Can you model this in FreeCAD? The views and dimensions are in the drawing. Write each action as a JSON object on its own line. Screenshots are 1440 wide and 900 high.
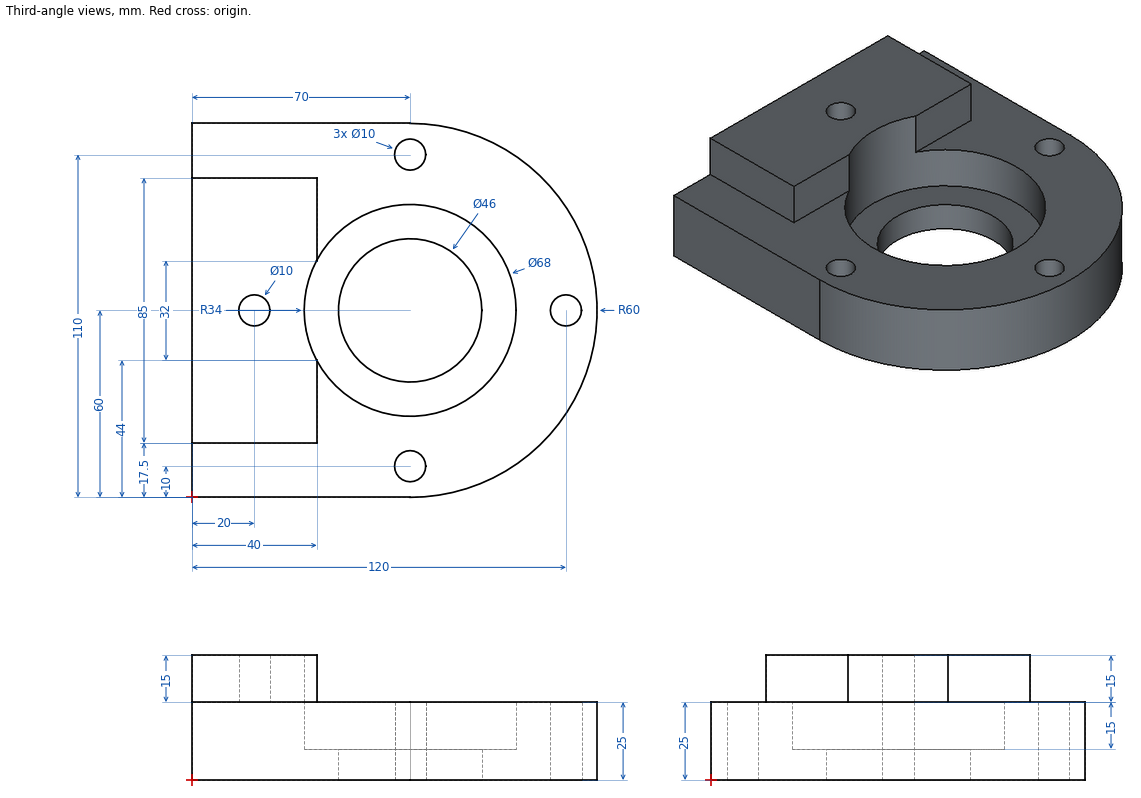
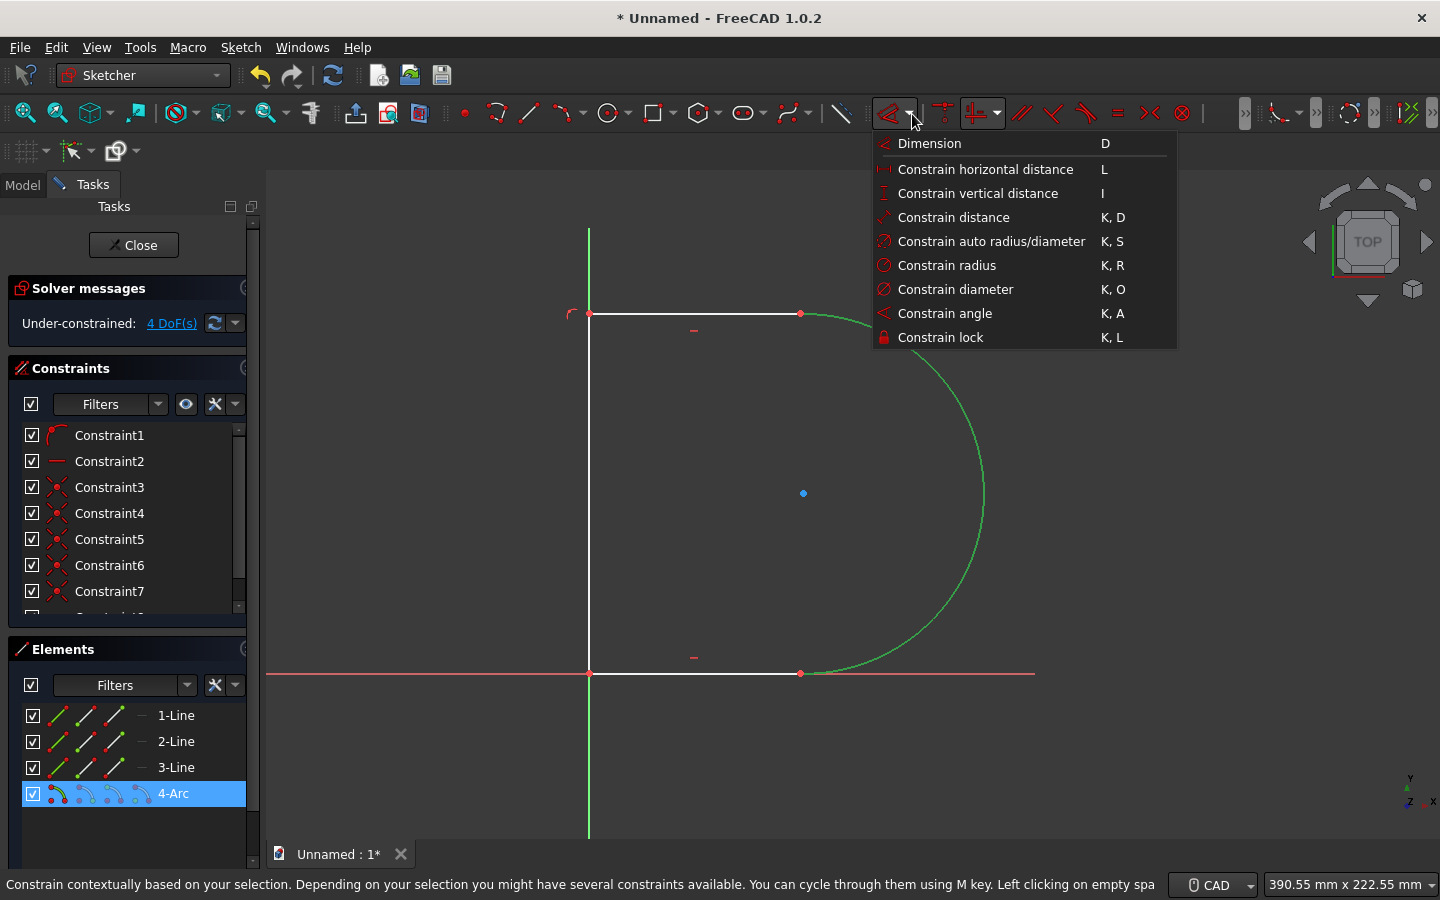
{"action": "left_click", "coordinate": [1025, 265]}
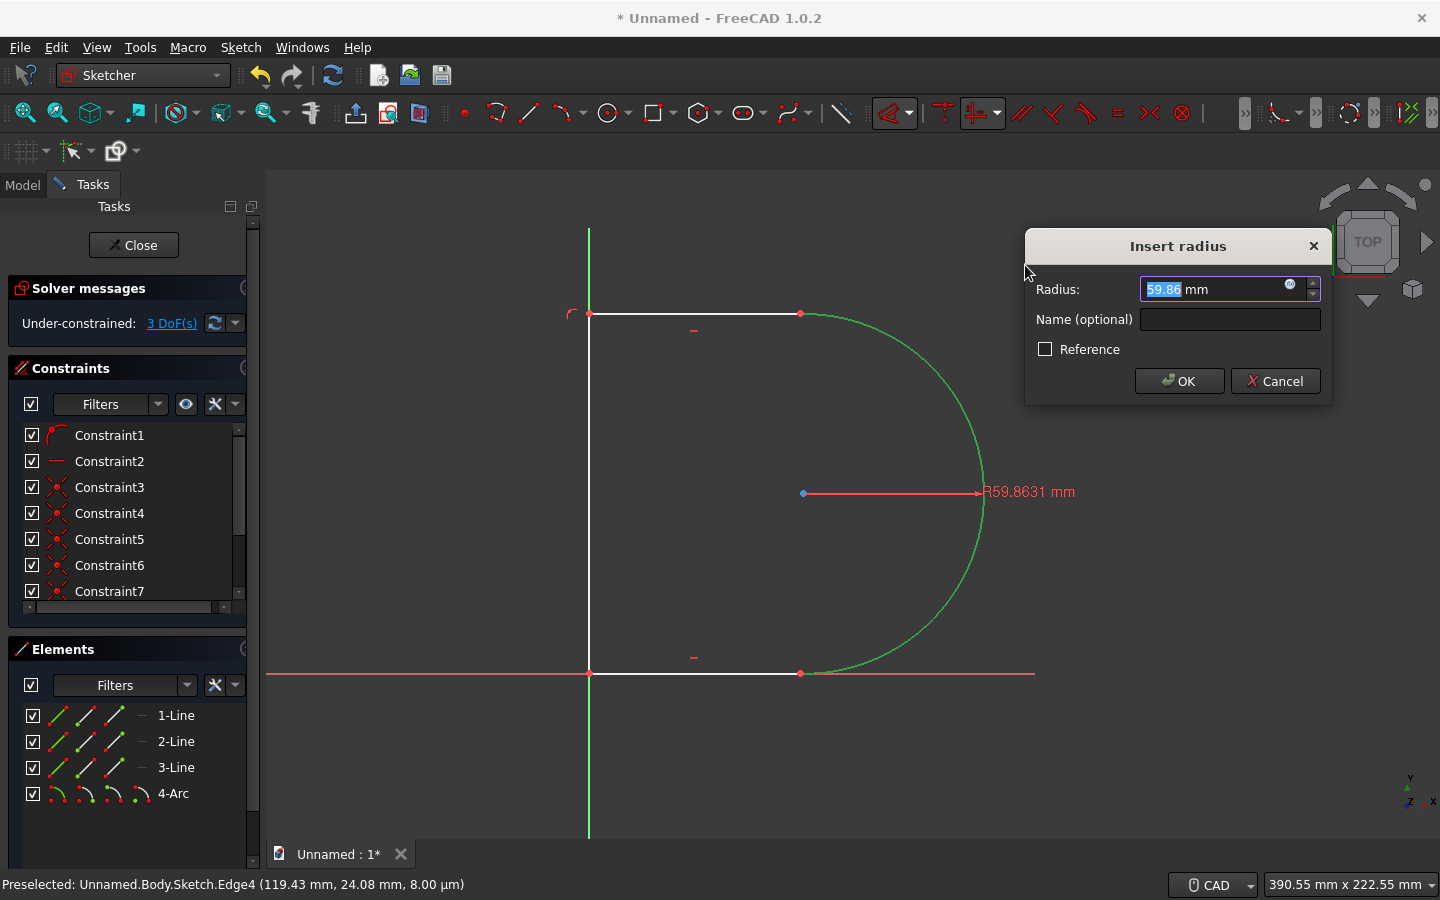
{"action": "type", "text": "60"}
{"action": "key", "text": "Return"}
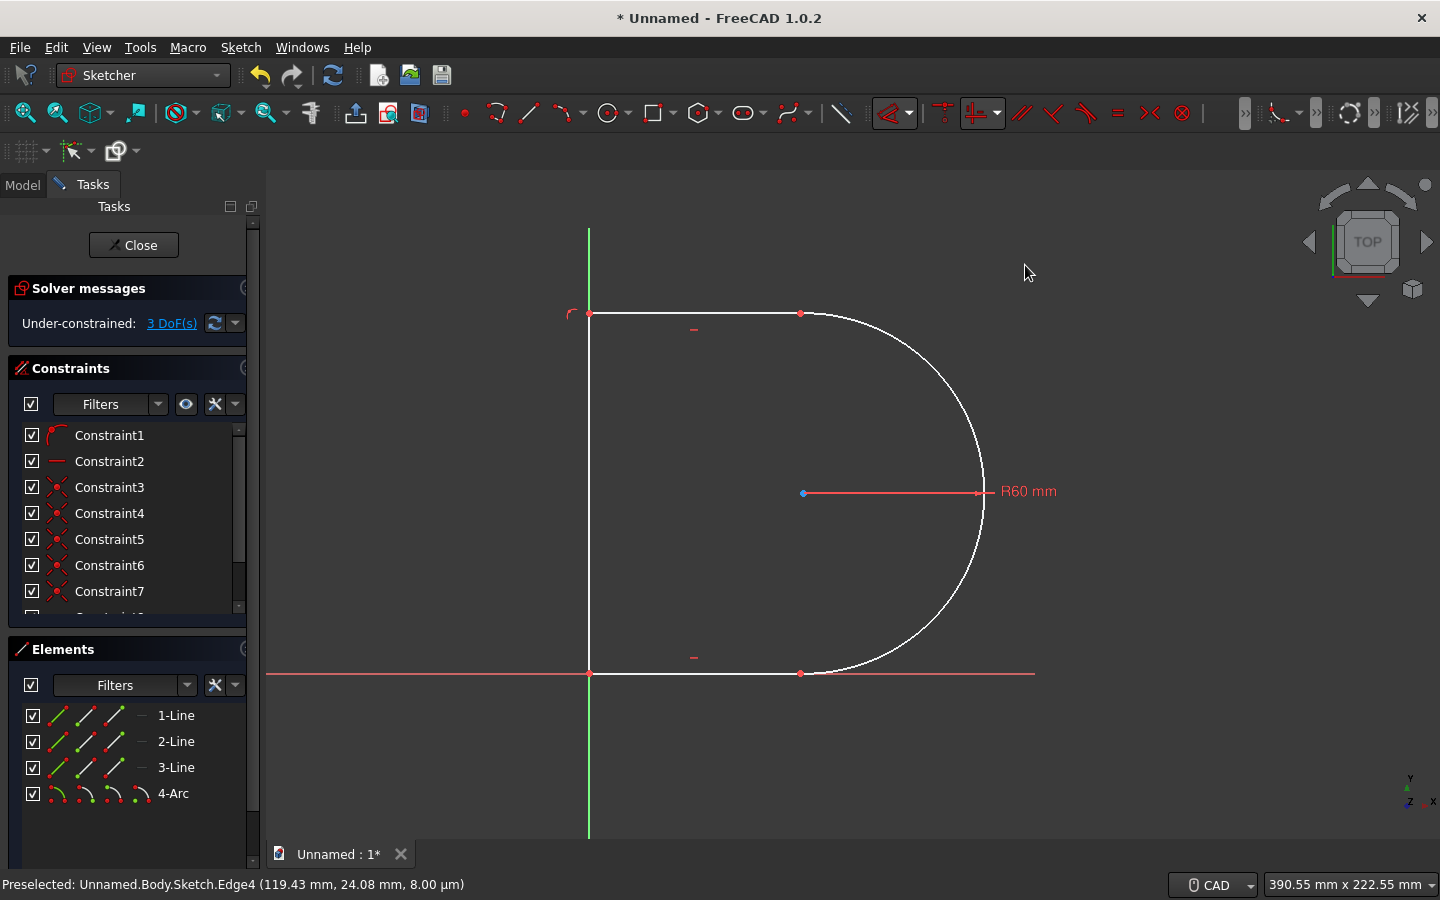
{"action": "left_click", "coordinate": [737, 313]}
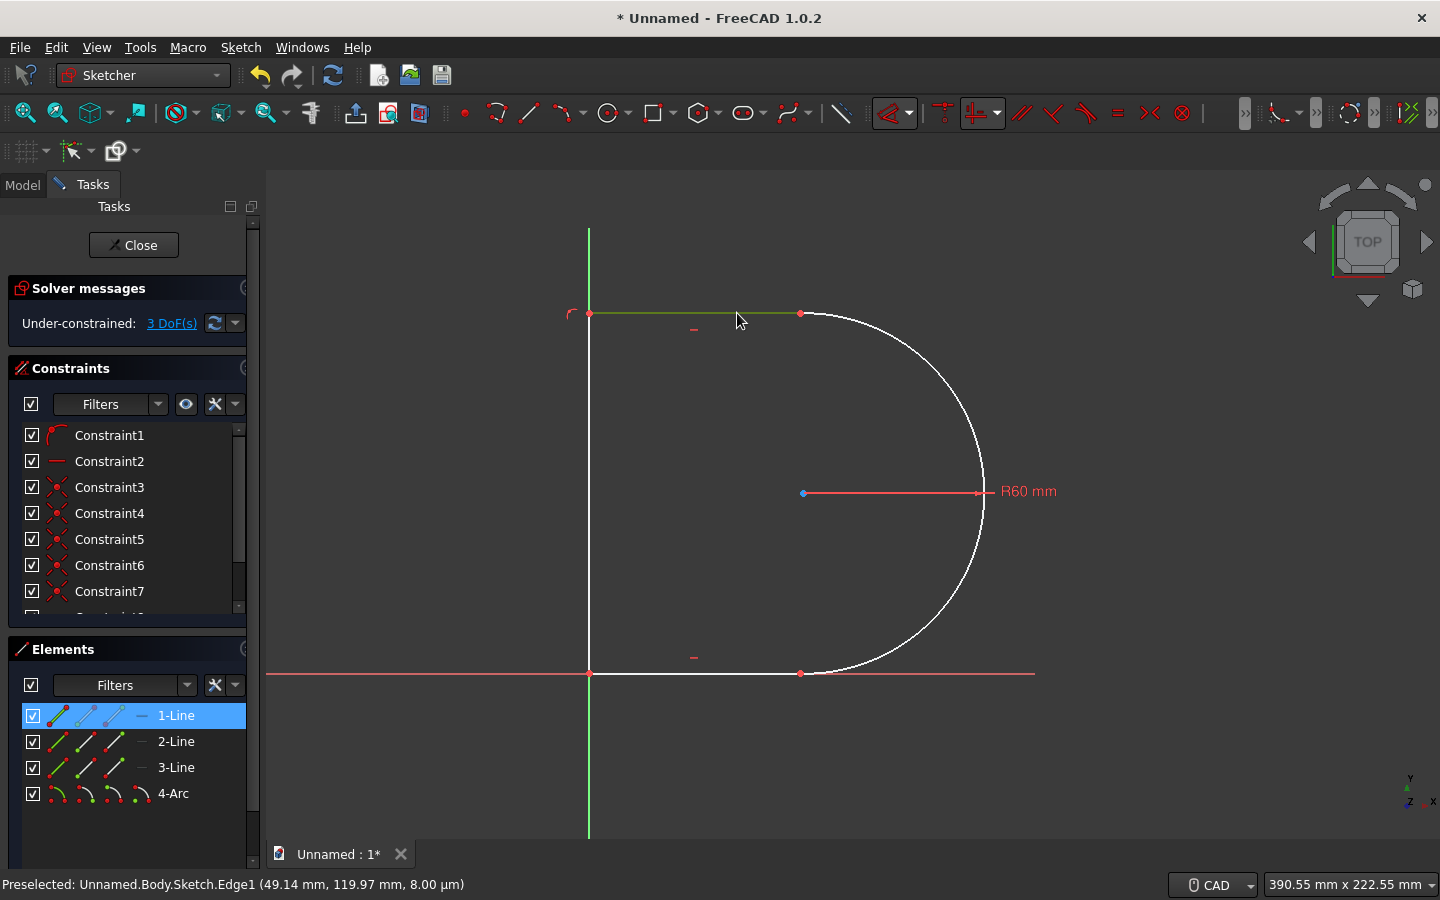
{"action": "left_click", "coordinate": [912, 114]}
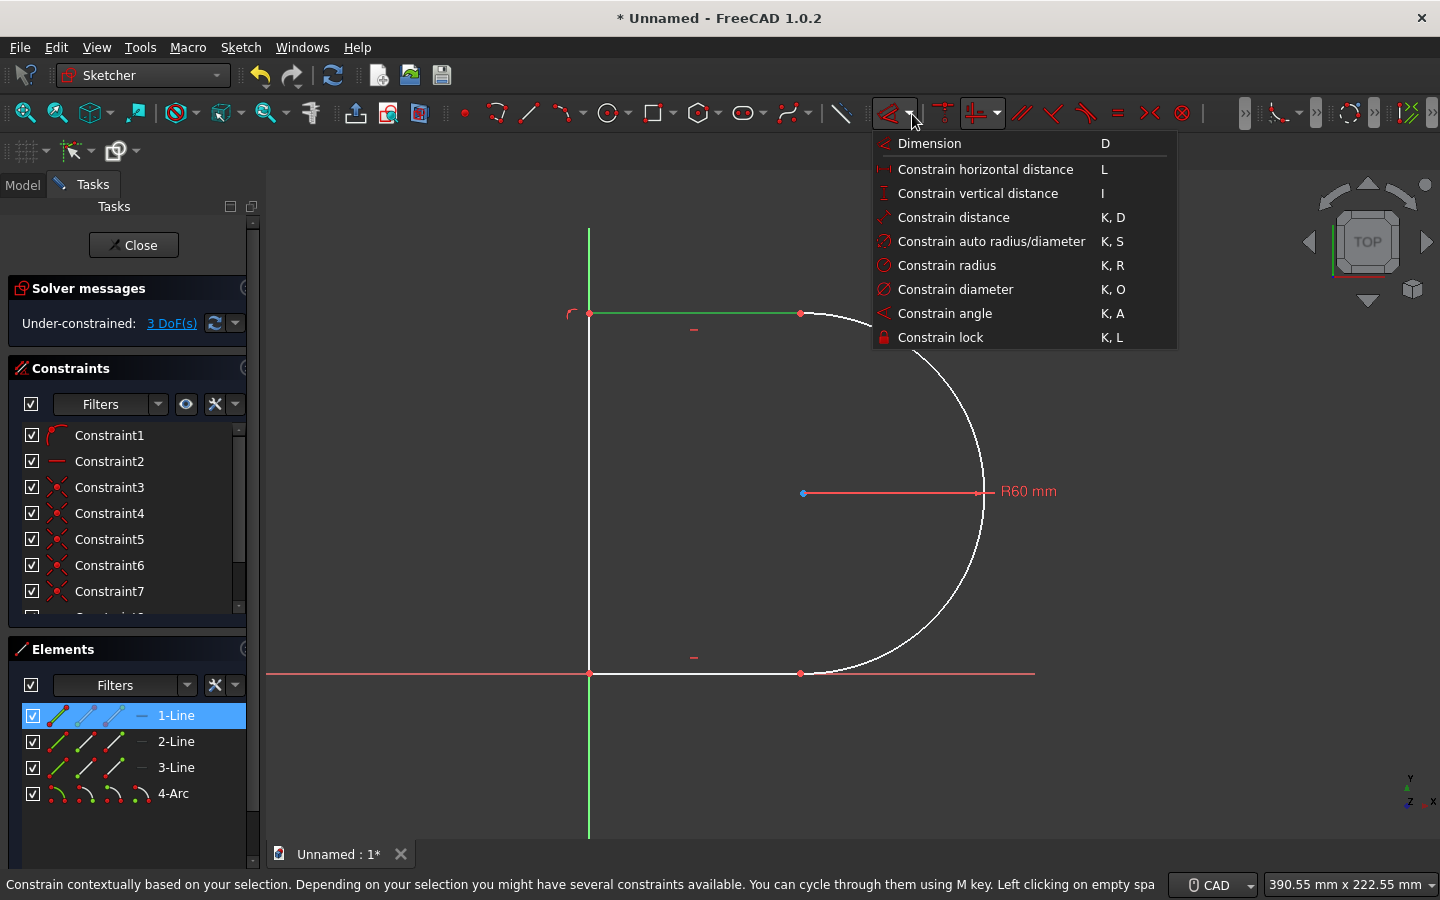
{"action": "left_click", "coordinate": [1025, 169]}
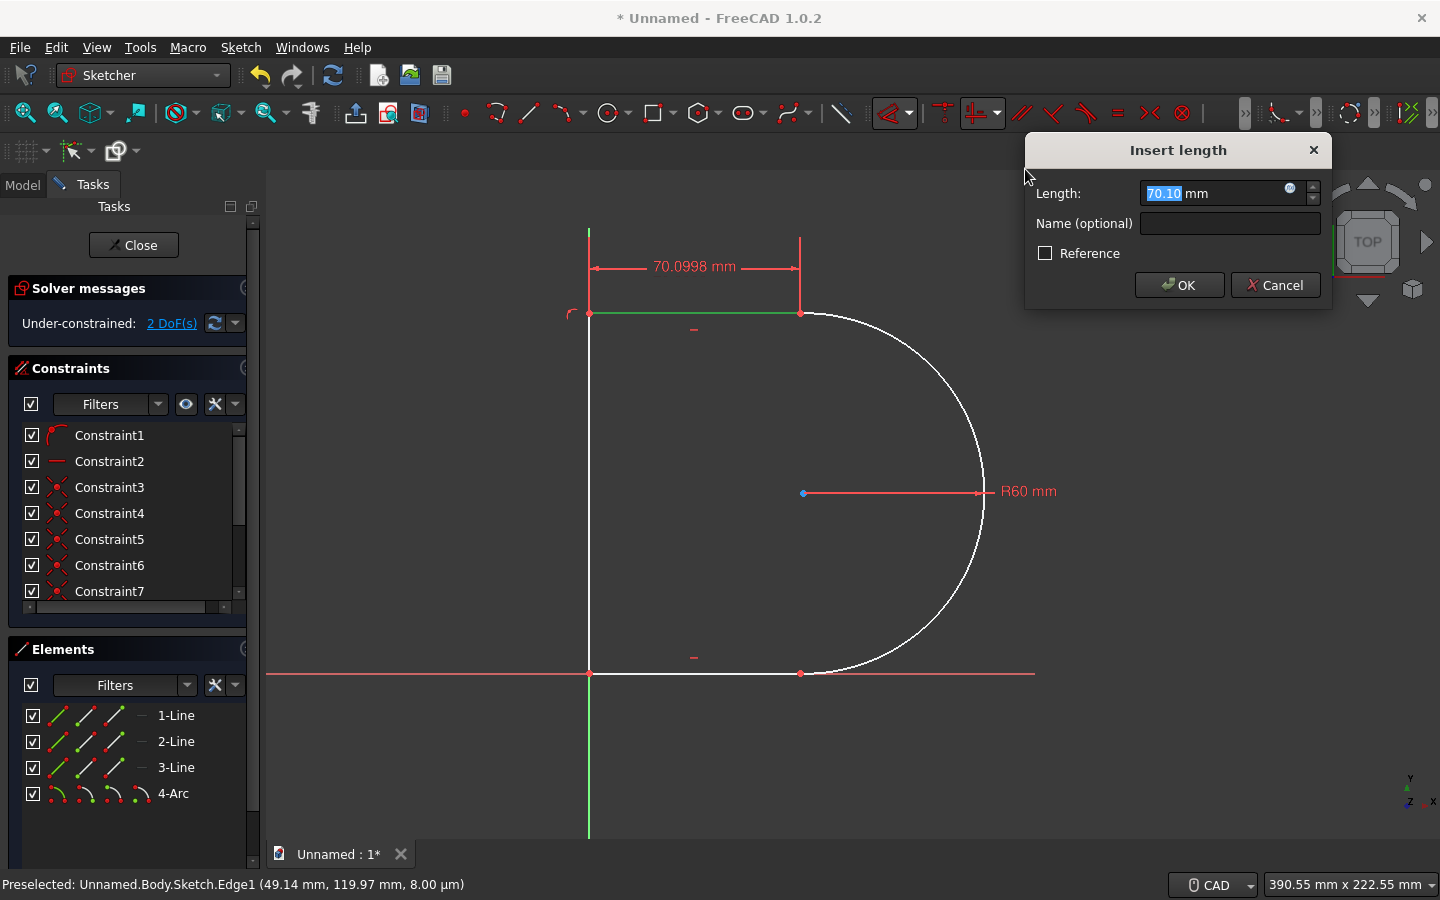
{"action": "type", "text": "70"}
{"action": "key", "text": "Return"}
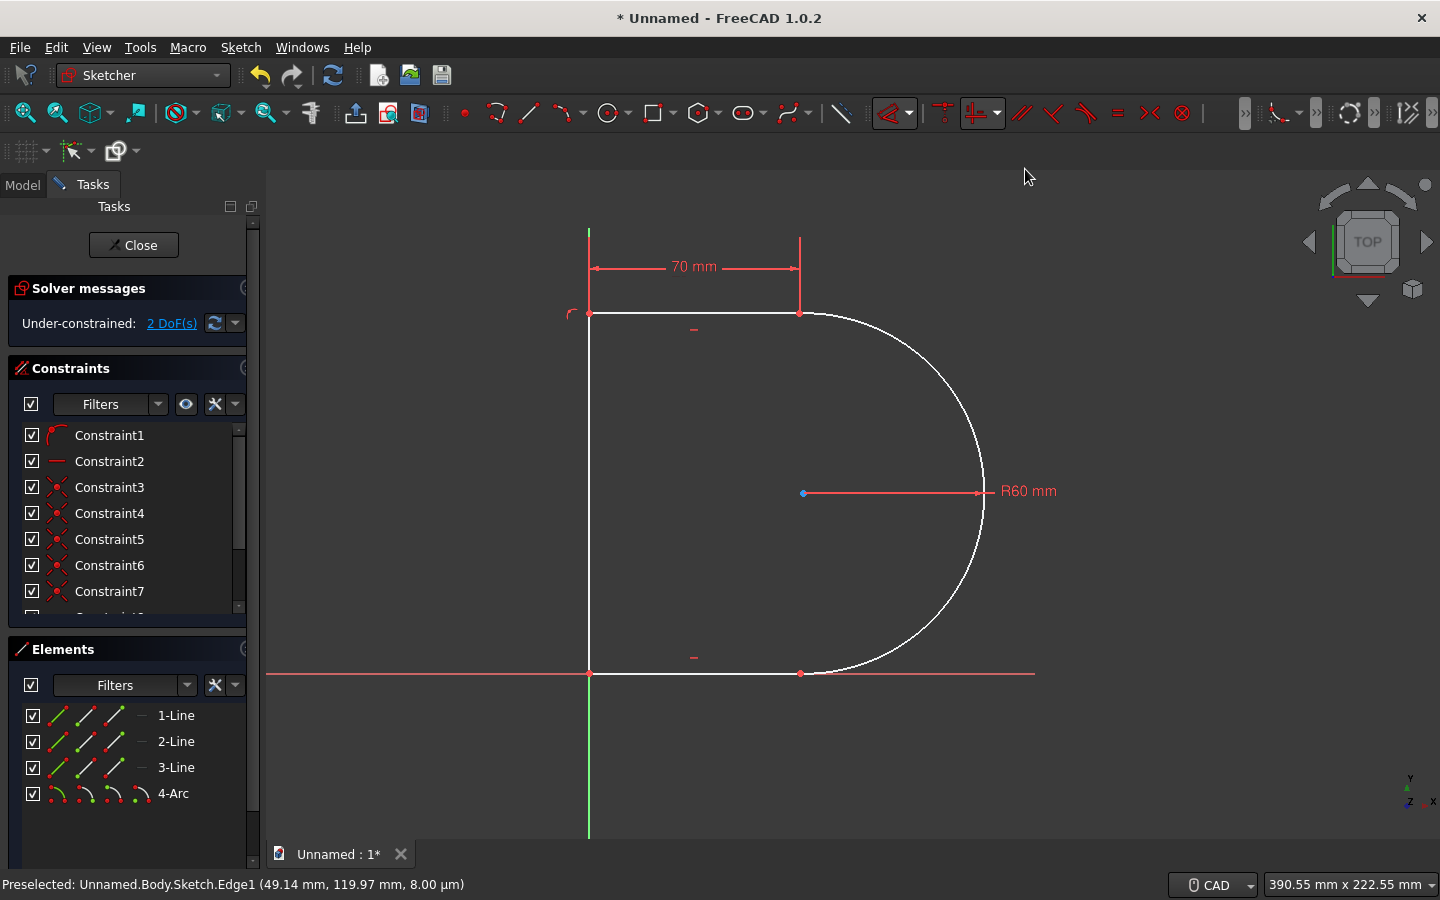
{"action": "left_click", "coordinate": [652, 674]}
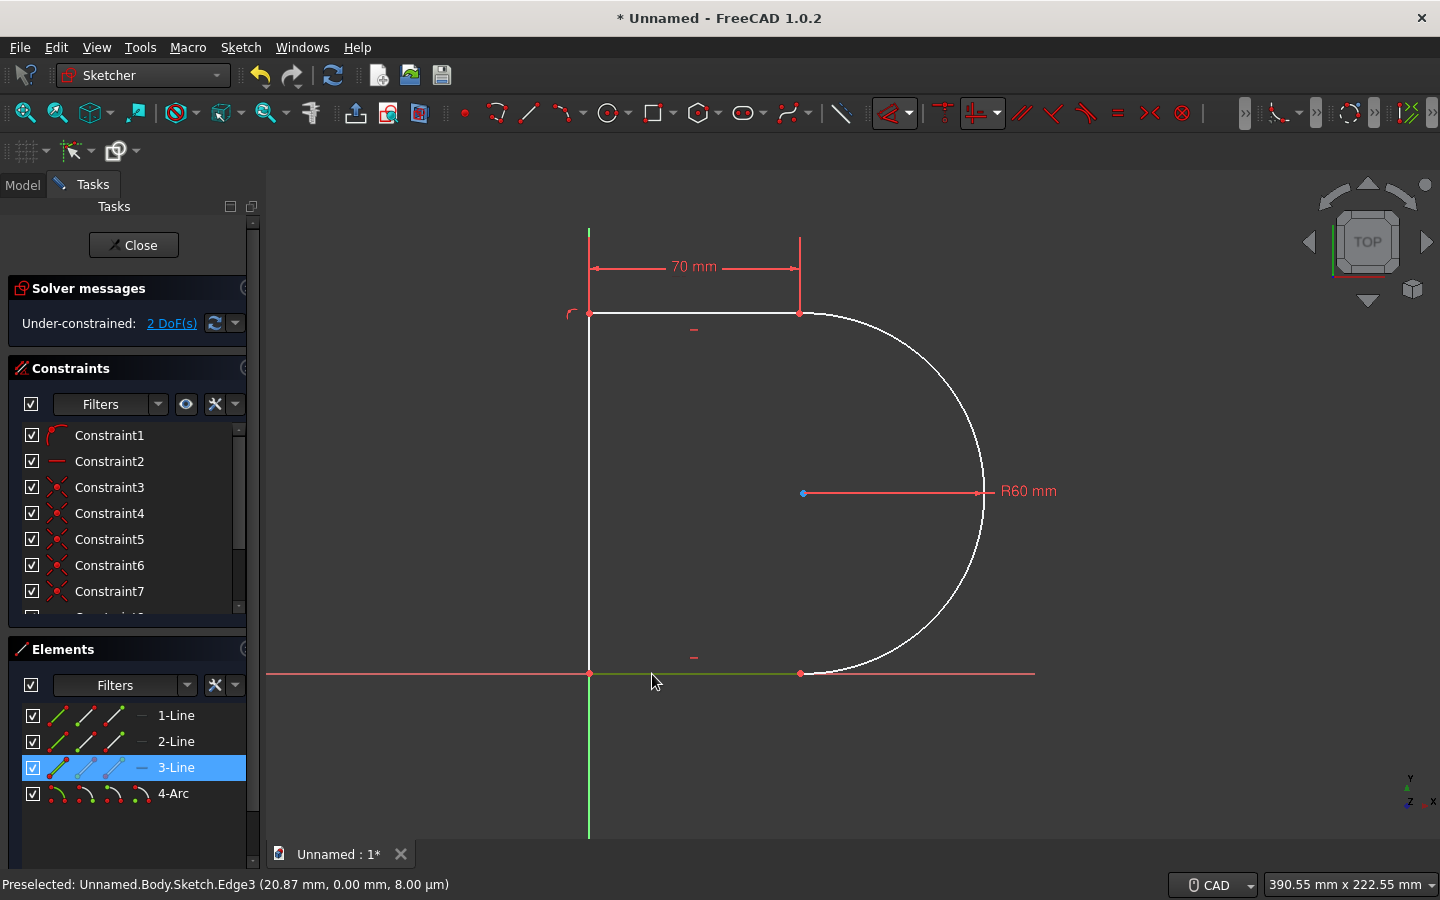
{"action": "key", "text": "l"}